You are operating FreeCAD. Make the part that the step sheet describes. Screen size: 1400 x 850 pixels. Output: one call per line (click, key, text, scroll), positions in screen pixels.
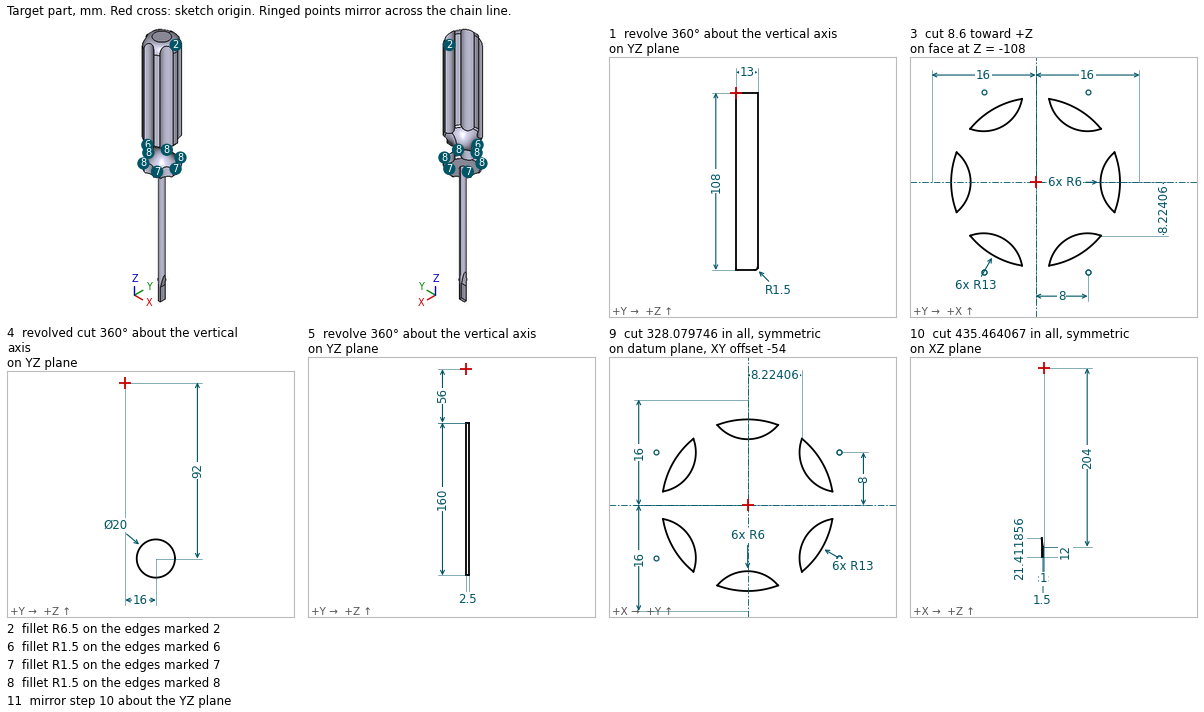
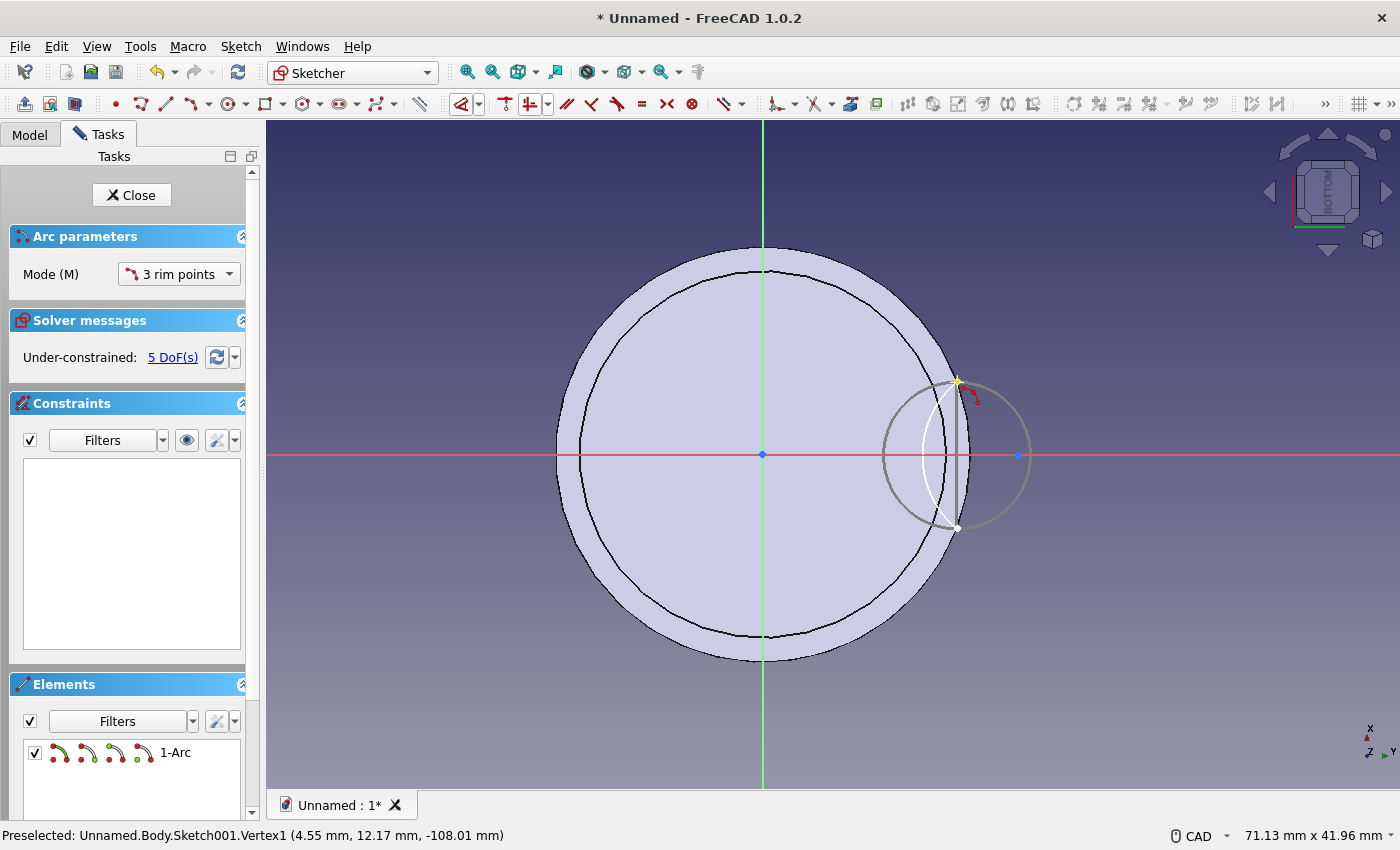
scroll(970, 470, up, 2)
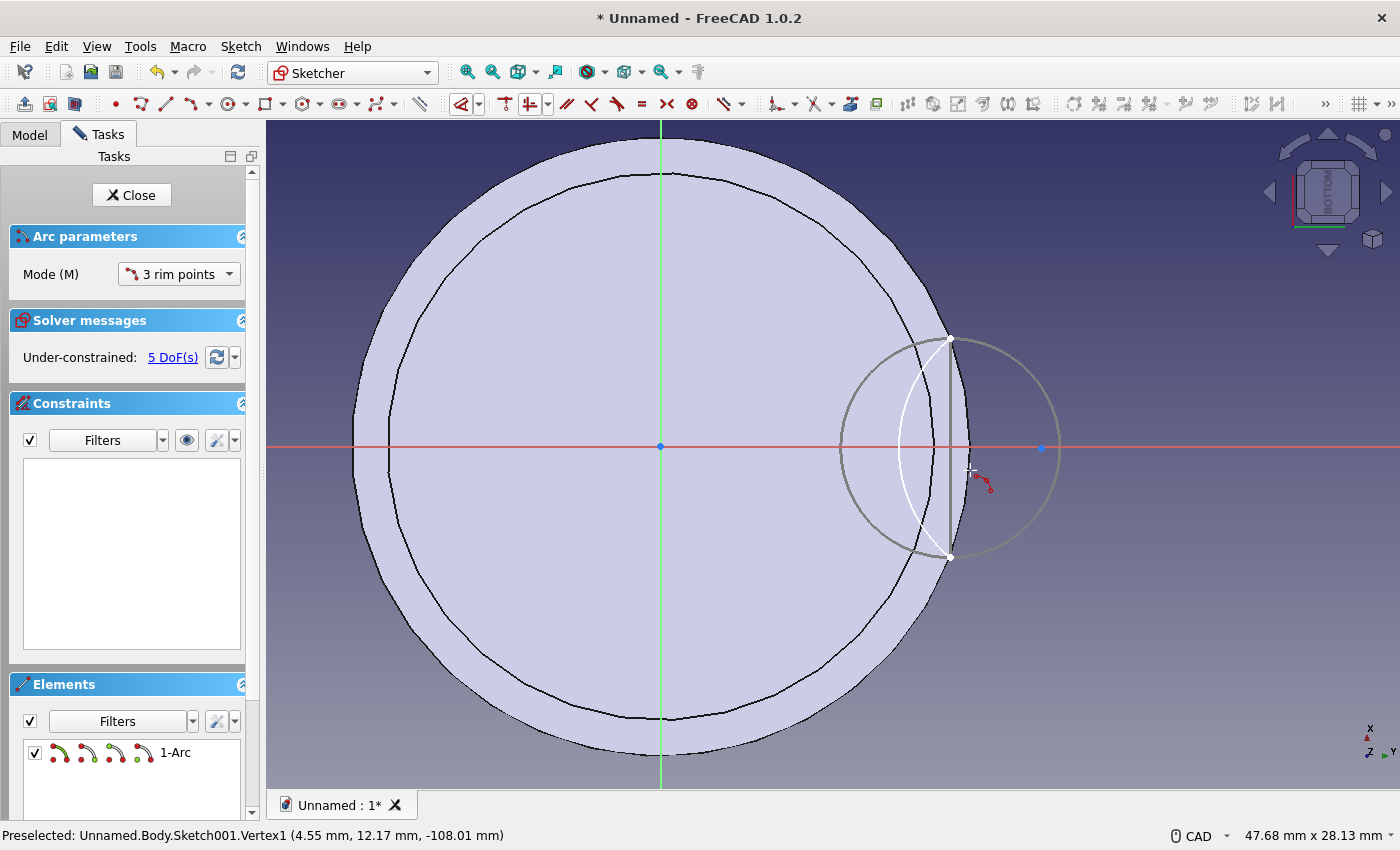
click(969, 469)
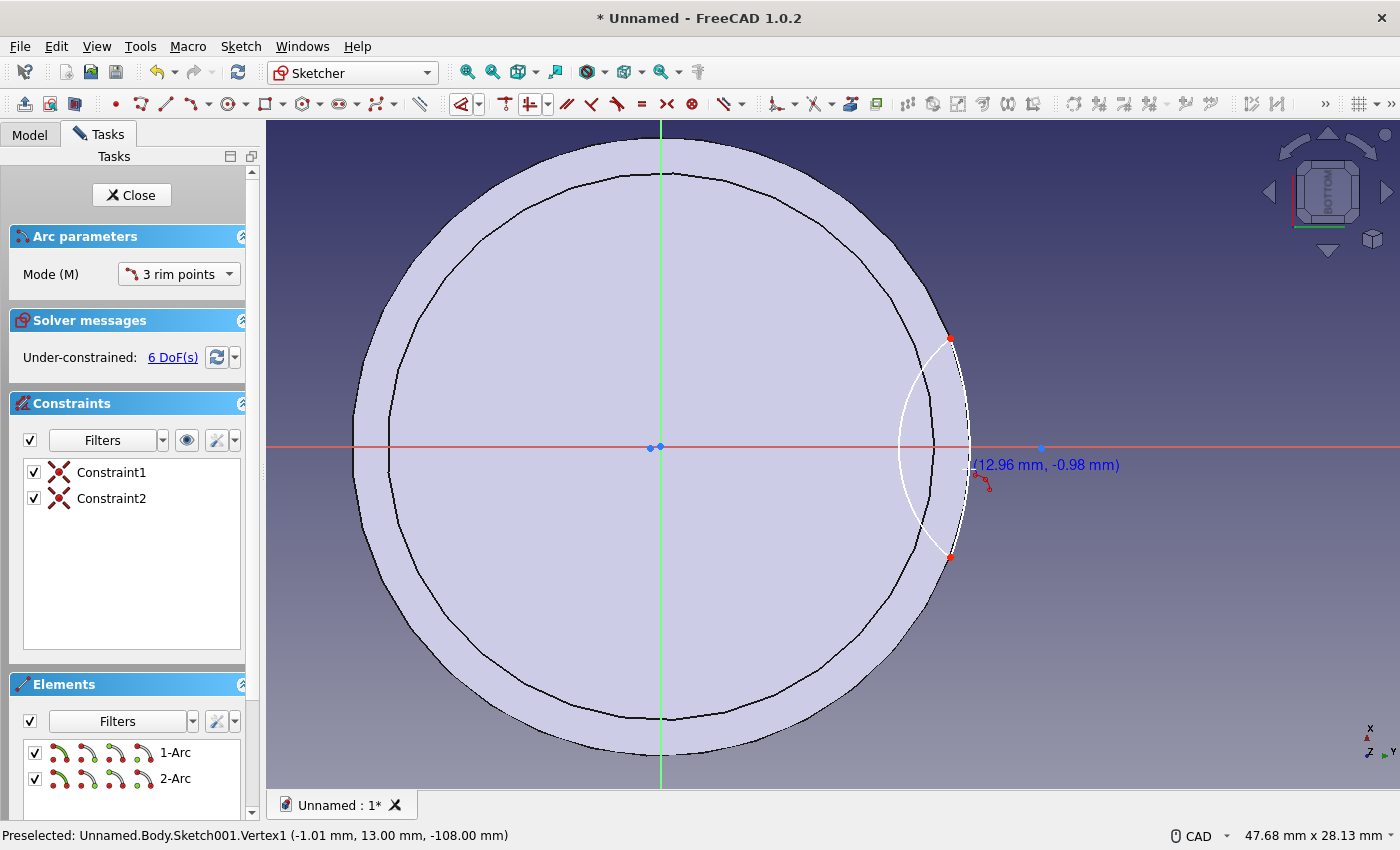
click(710, 752)
click(900, 642)
click(815, 714)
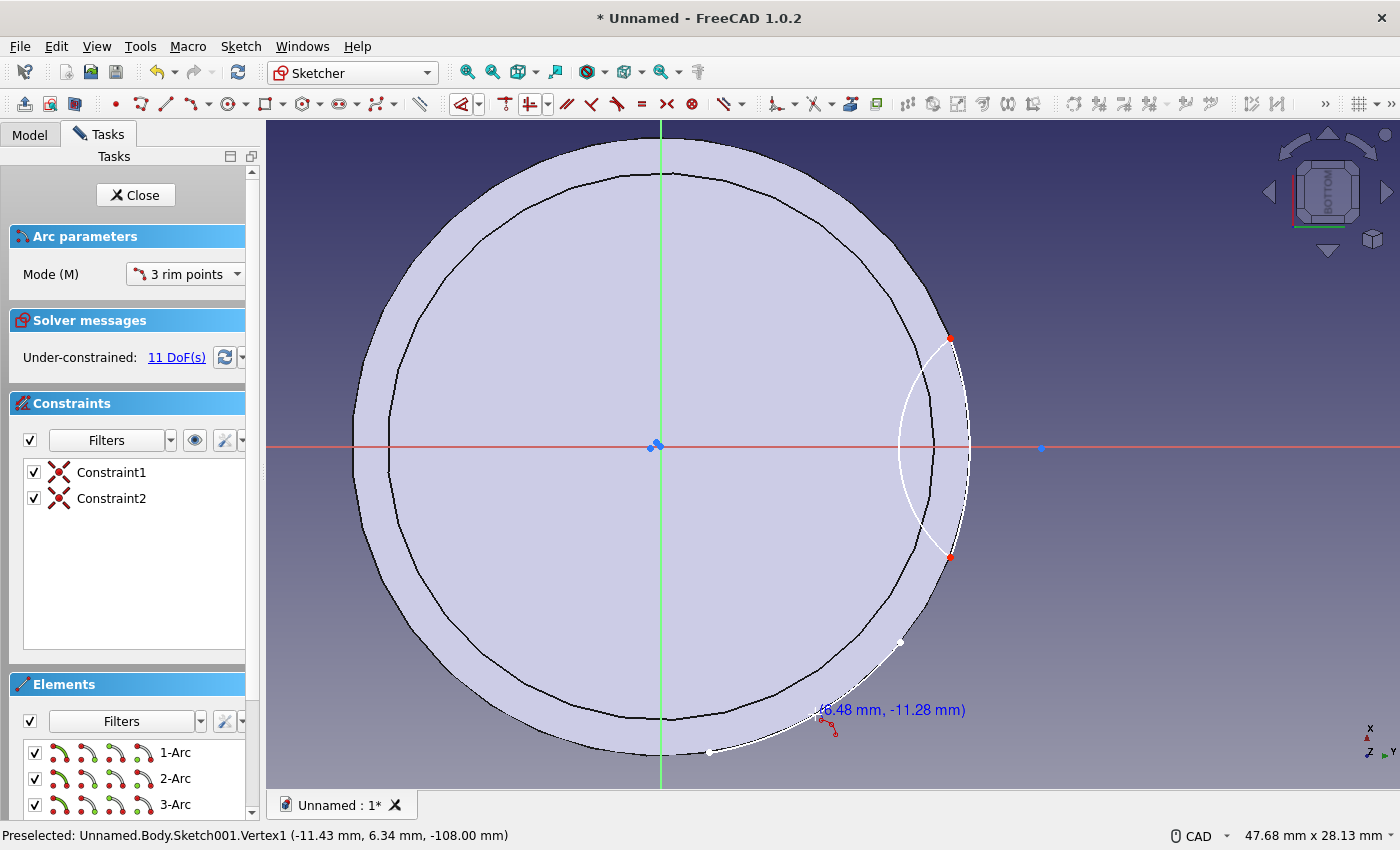
click(900, 643)
click(710, 753)
click(780, 653)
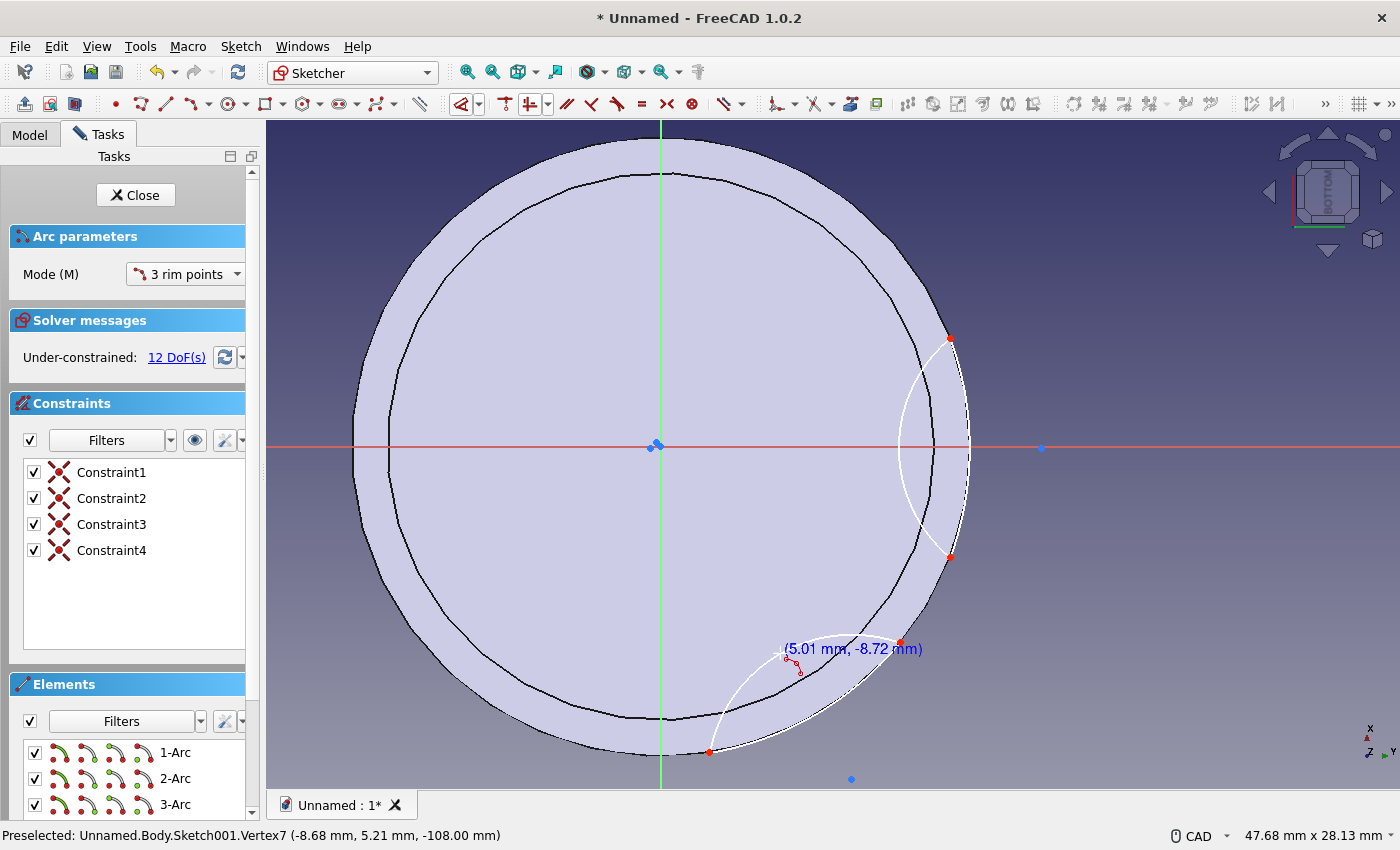
click(611, 752)
click(421, 642)
click(542, 653)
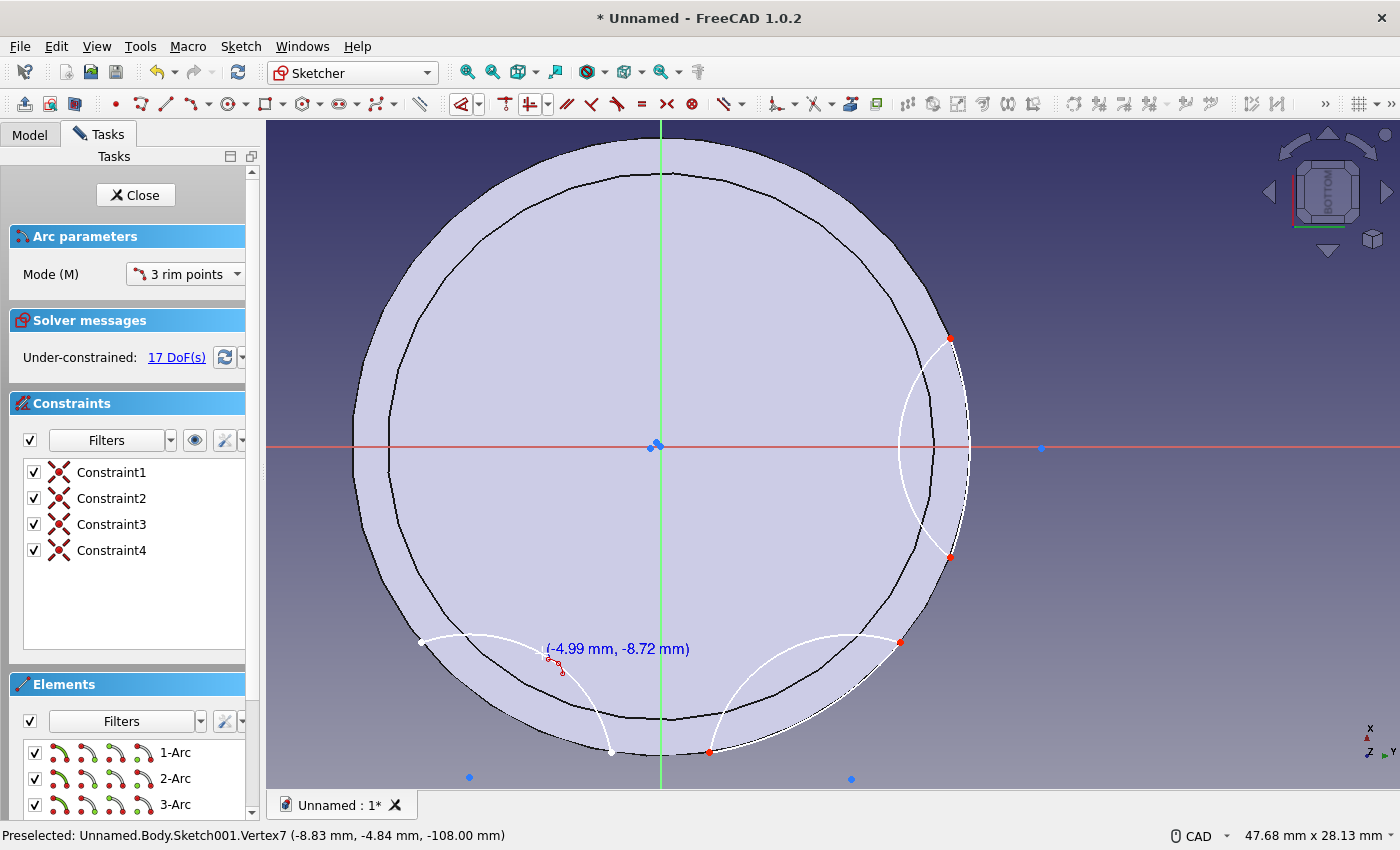
click(421, 643)
click(611, 753)
click(506, 714)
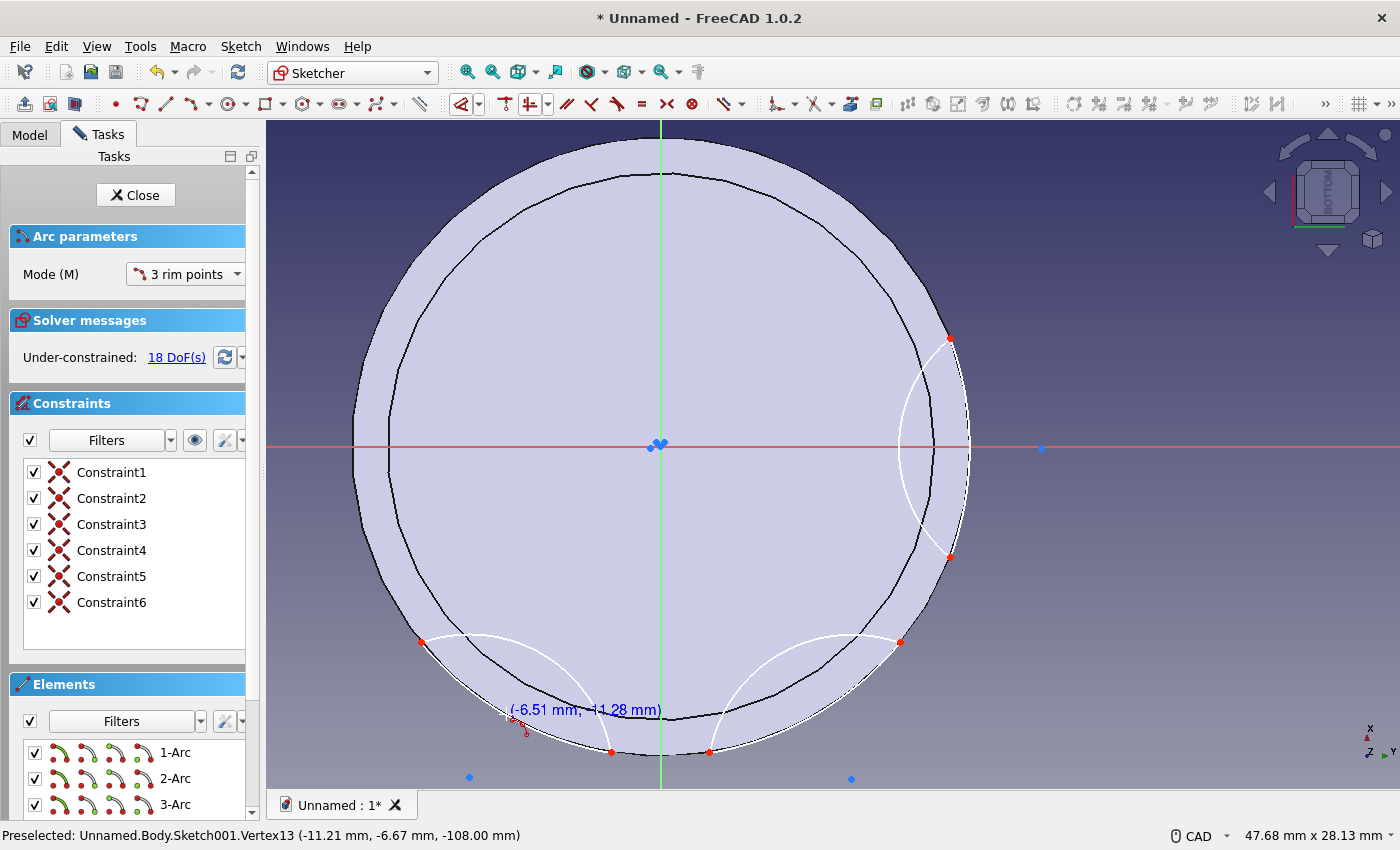
click(372, 556)
click(372, 337)
click(421, 471)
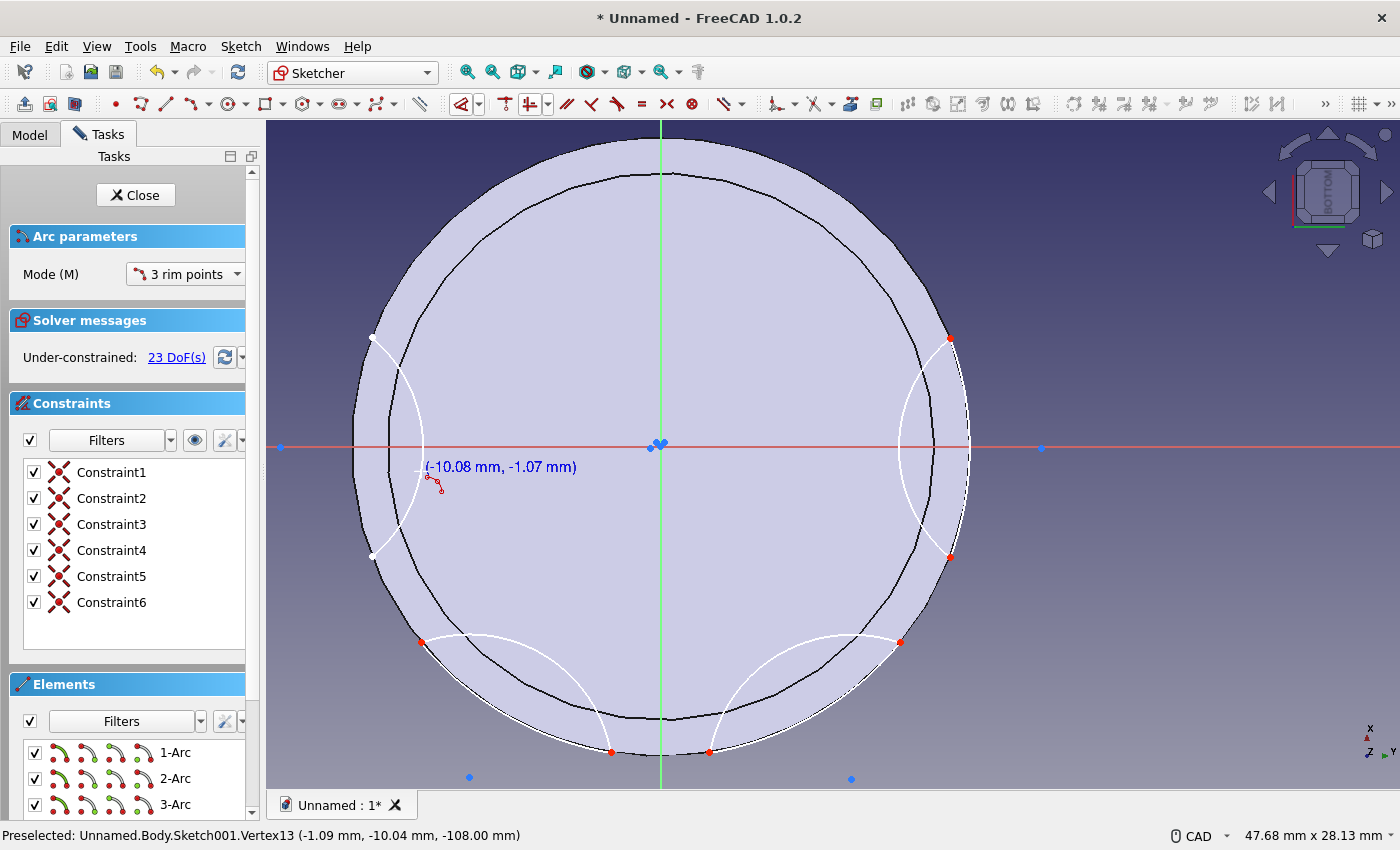
click(372, 338)
click(372, 557)
click(352, 424)